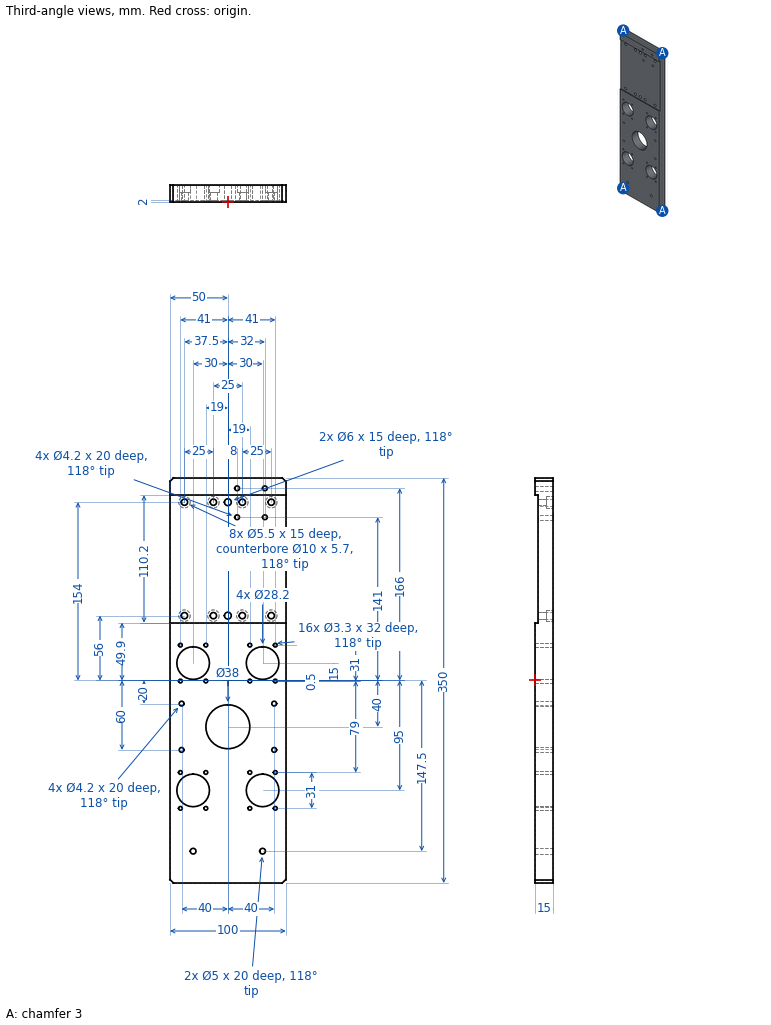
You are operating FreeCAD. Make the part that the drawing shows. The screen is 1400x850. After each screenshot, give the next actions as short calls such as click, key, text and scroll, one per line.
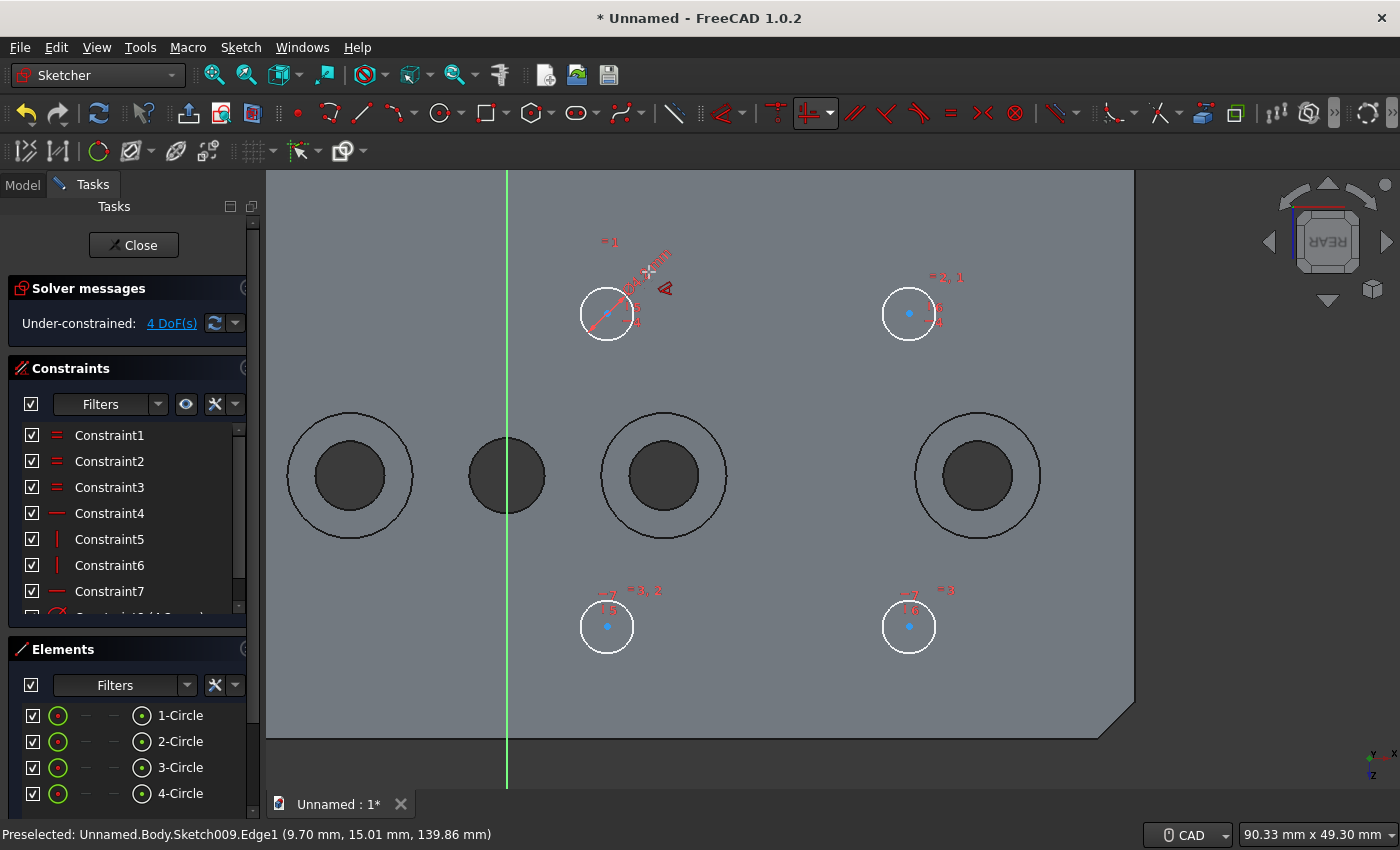
click(607, 314)
click(557, 348)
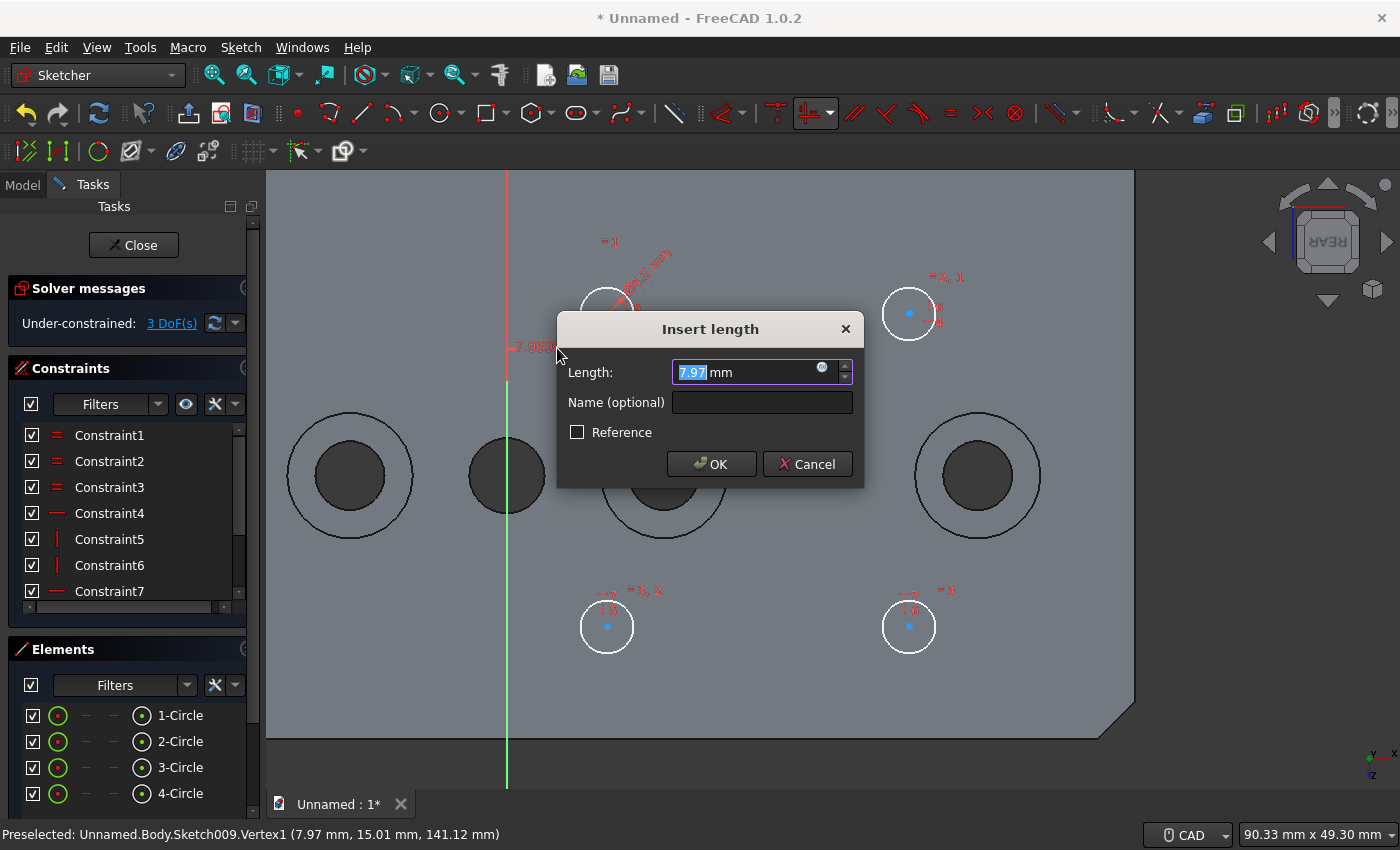
text(8)
key(Return)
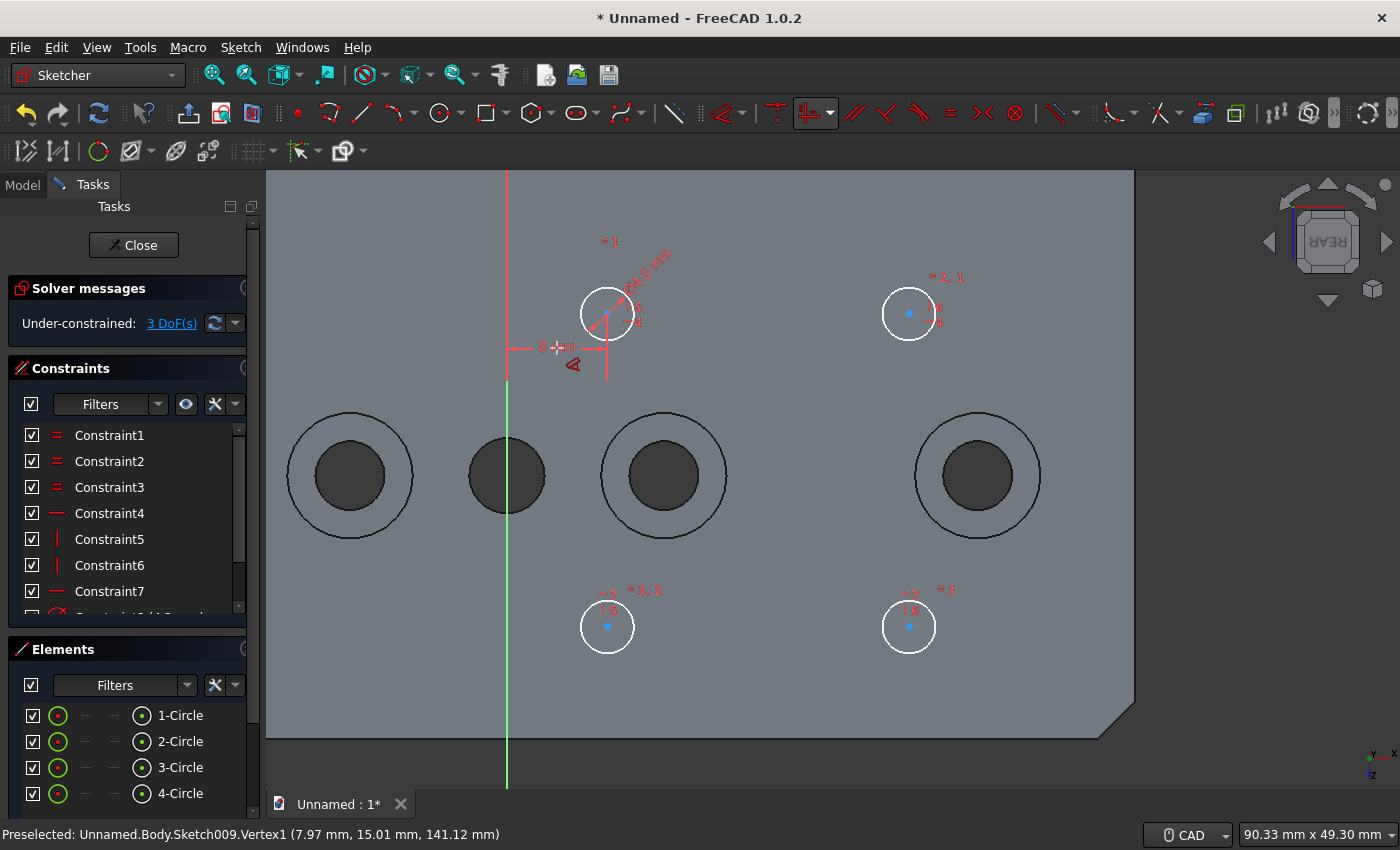
click(909, 314)
click(708, 348)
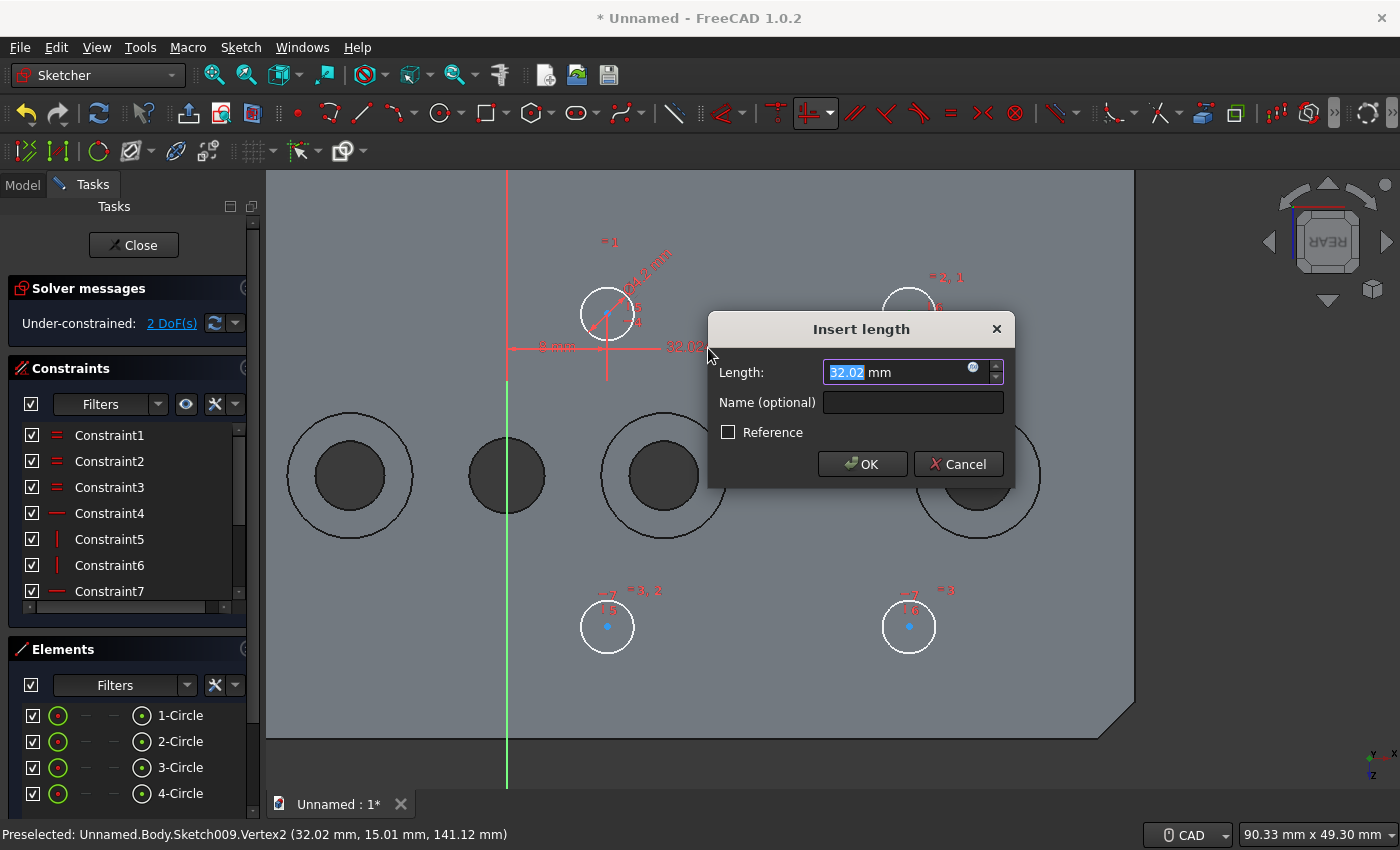
text(32)
key(Return)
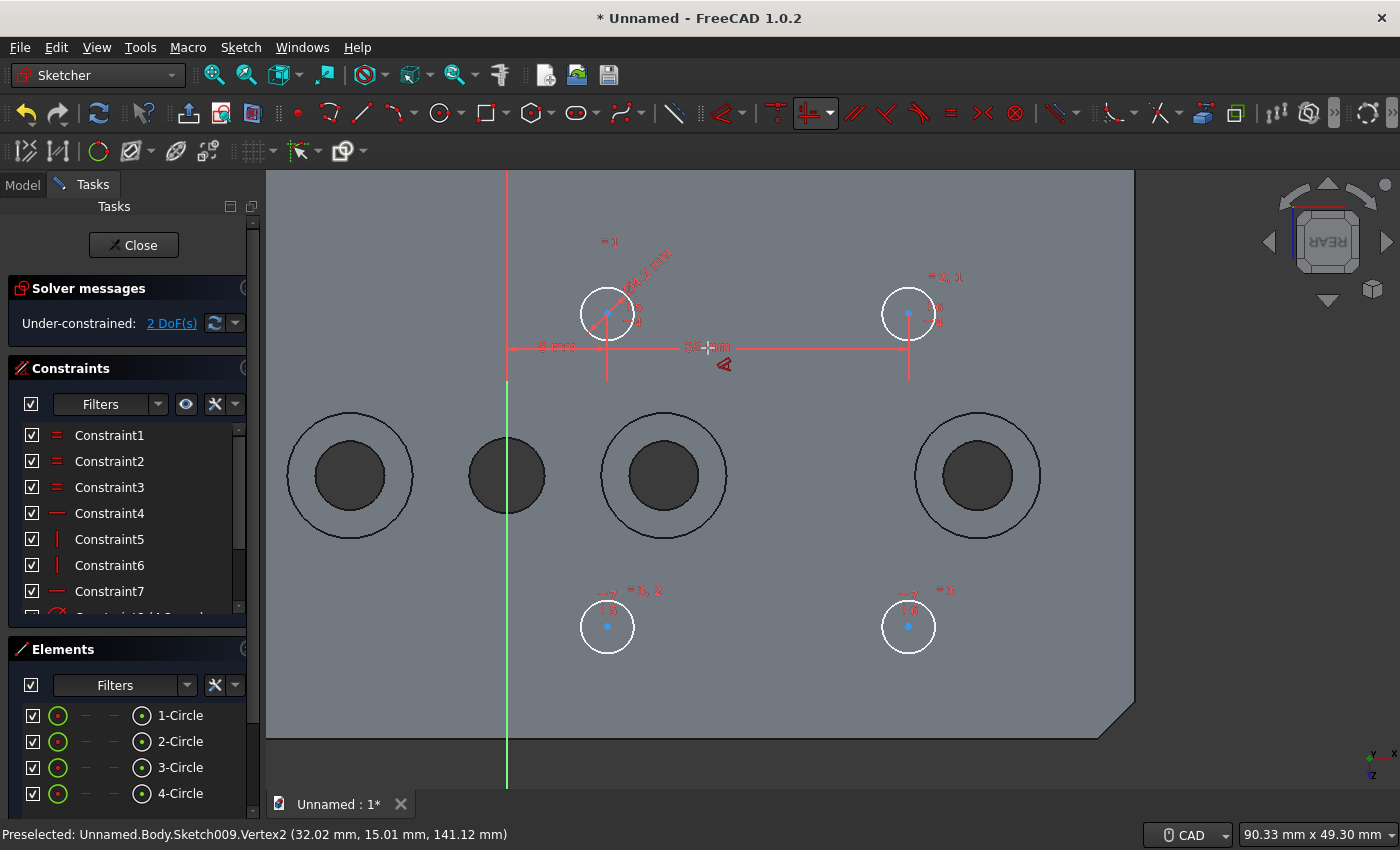
click(607, 314)
click(473, 256)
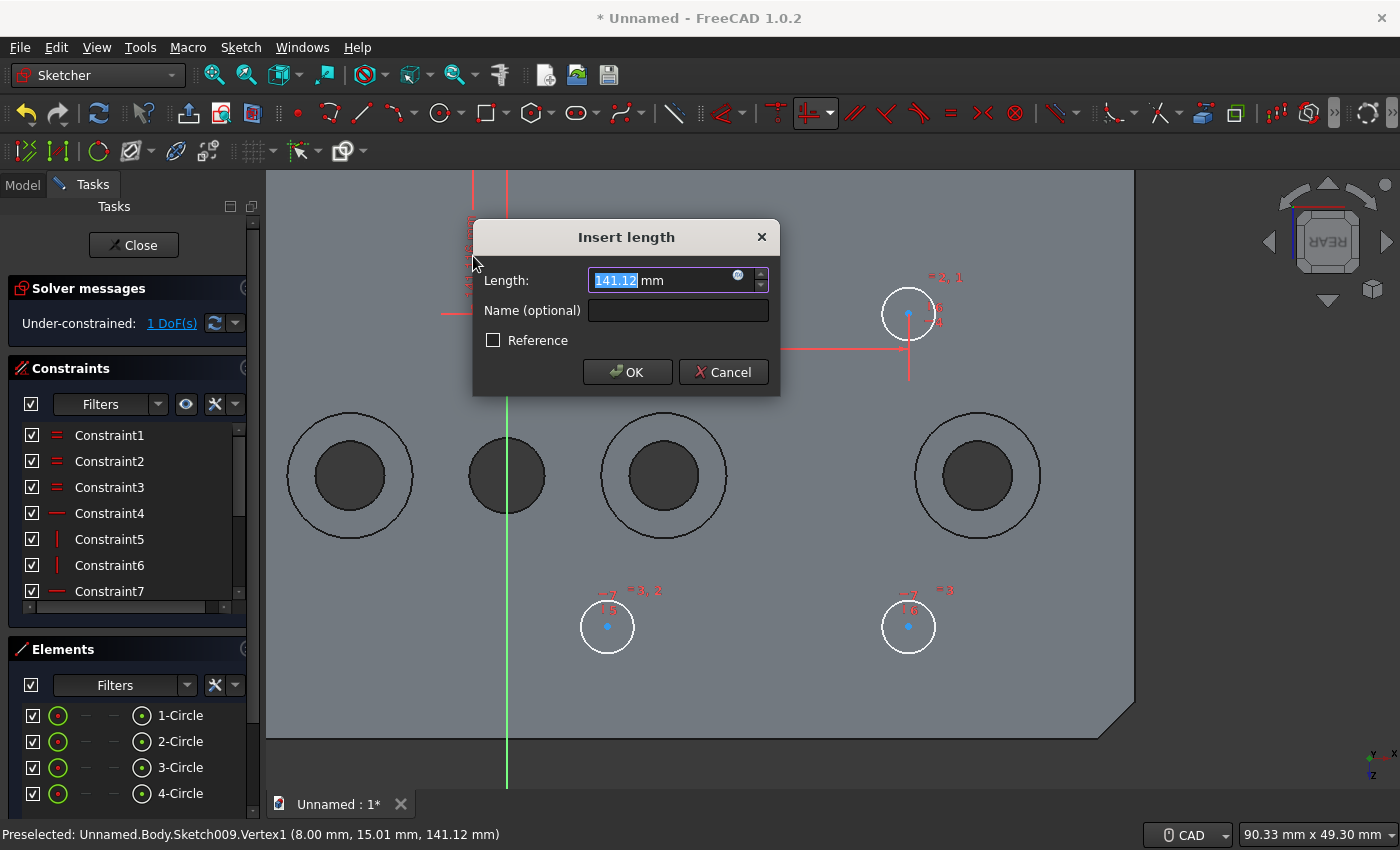
text(141)
key(Return)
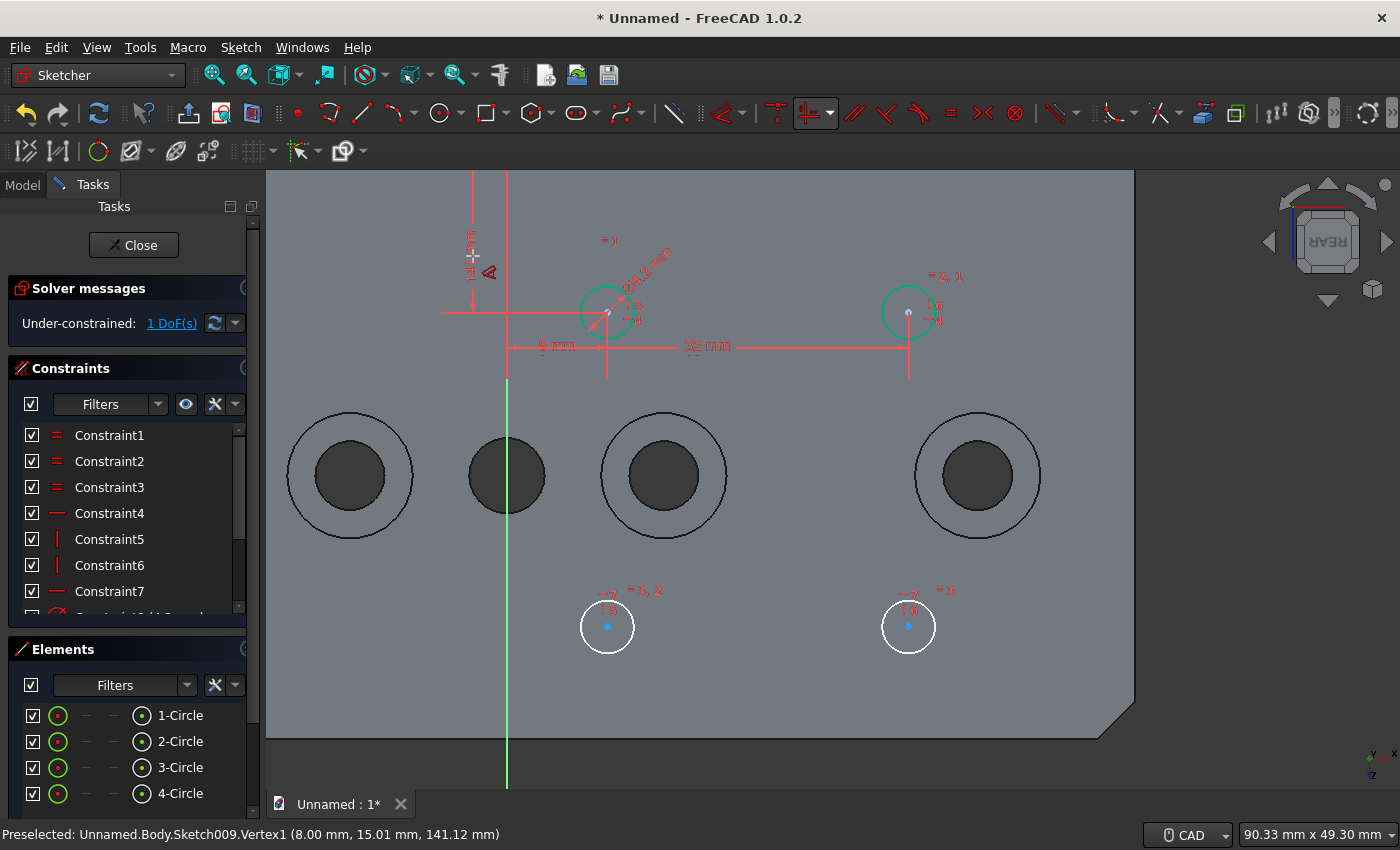
click(607, 627)
click(473, 412)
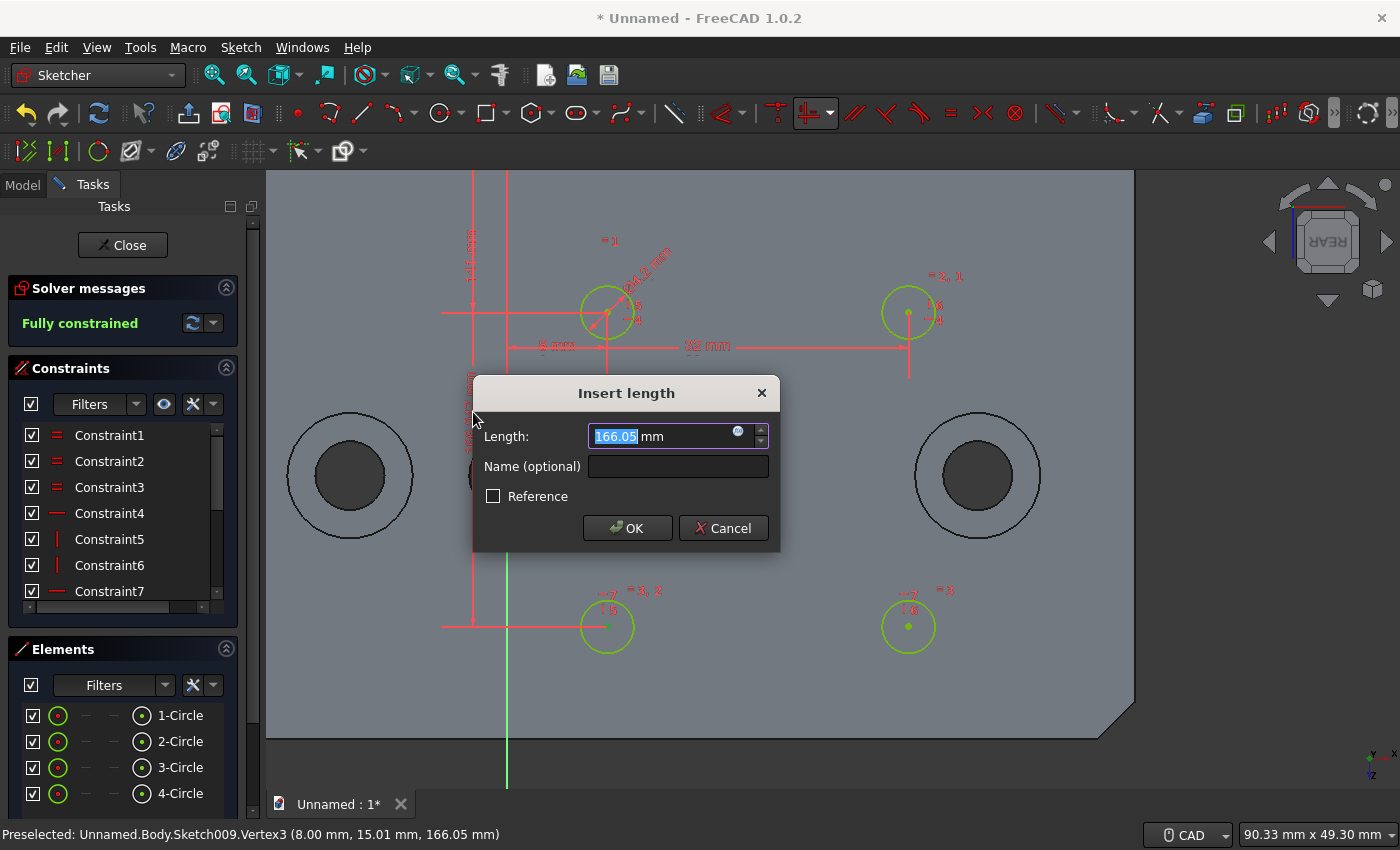
text(166)
key(Return)
key(Escape)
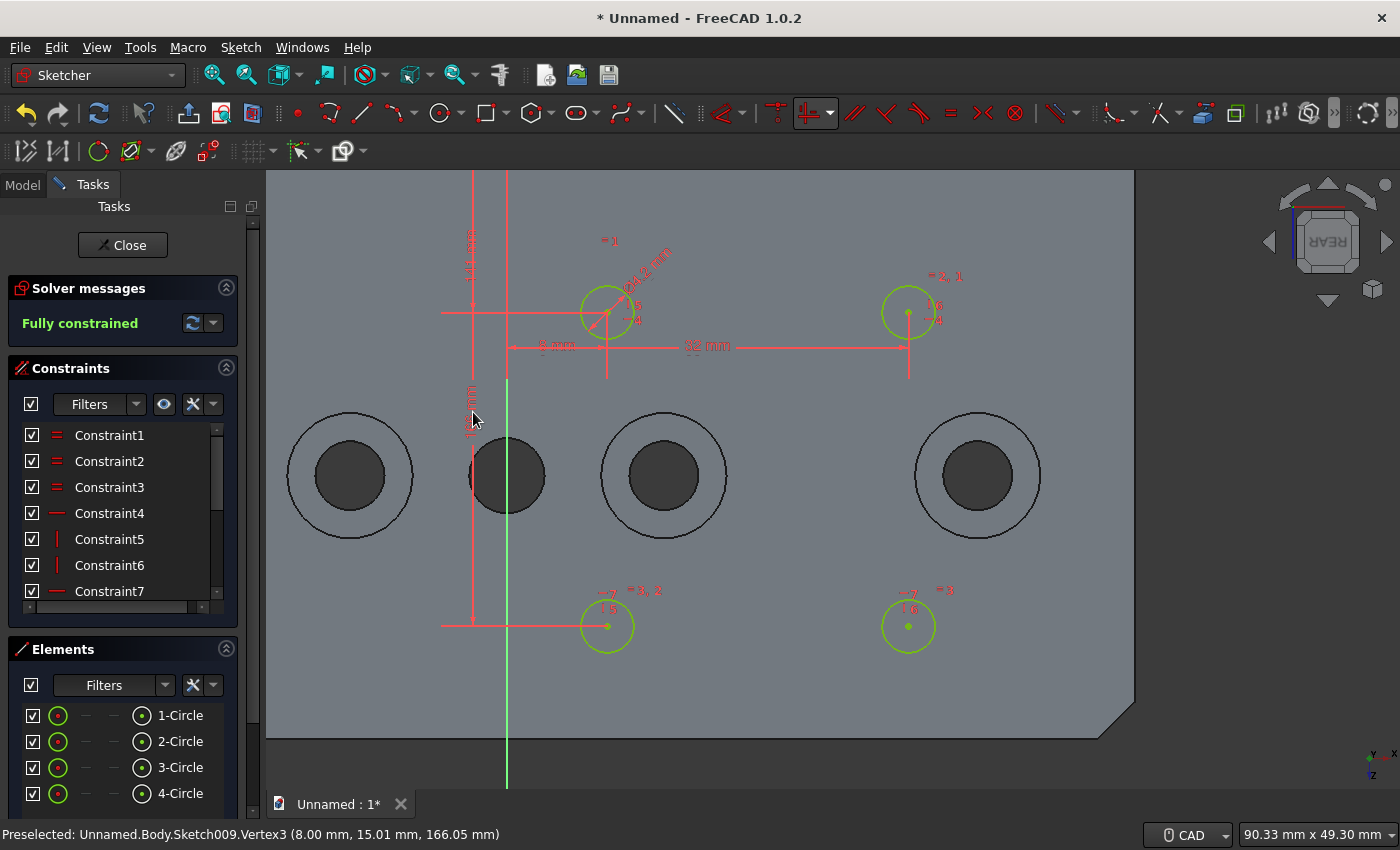
click(123, 245)